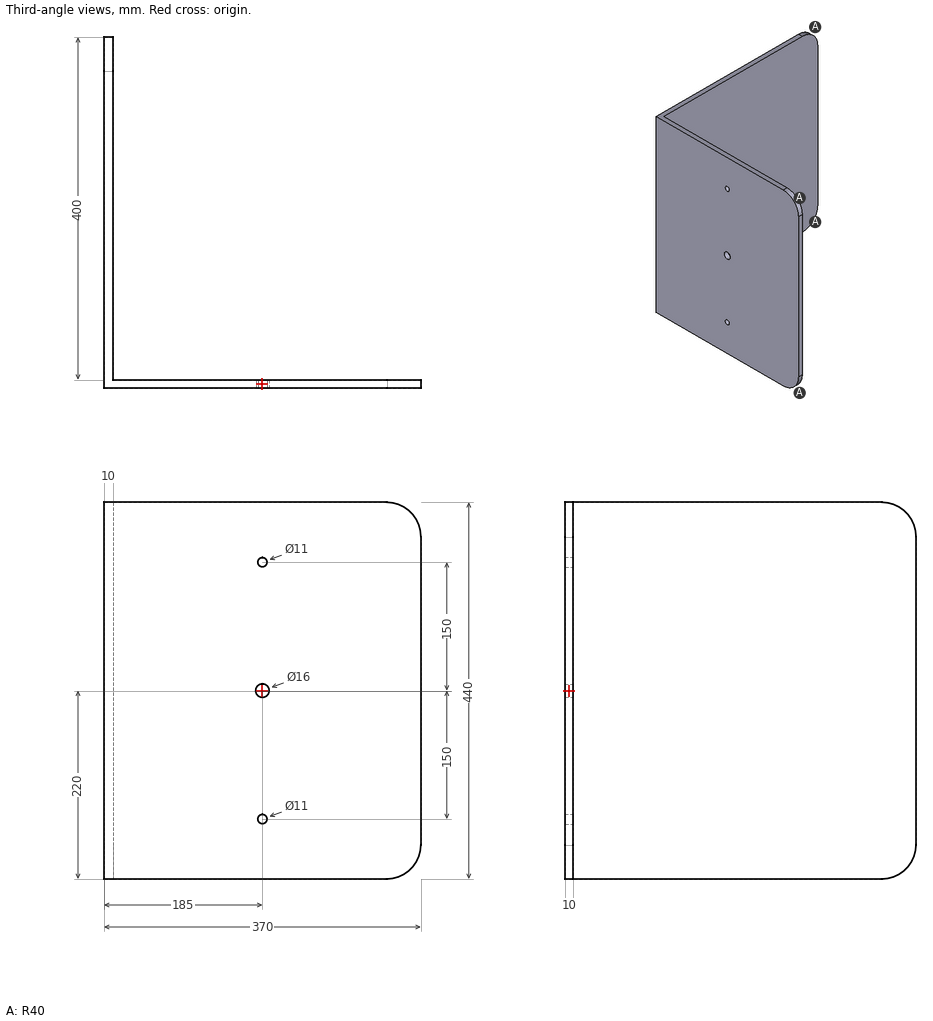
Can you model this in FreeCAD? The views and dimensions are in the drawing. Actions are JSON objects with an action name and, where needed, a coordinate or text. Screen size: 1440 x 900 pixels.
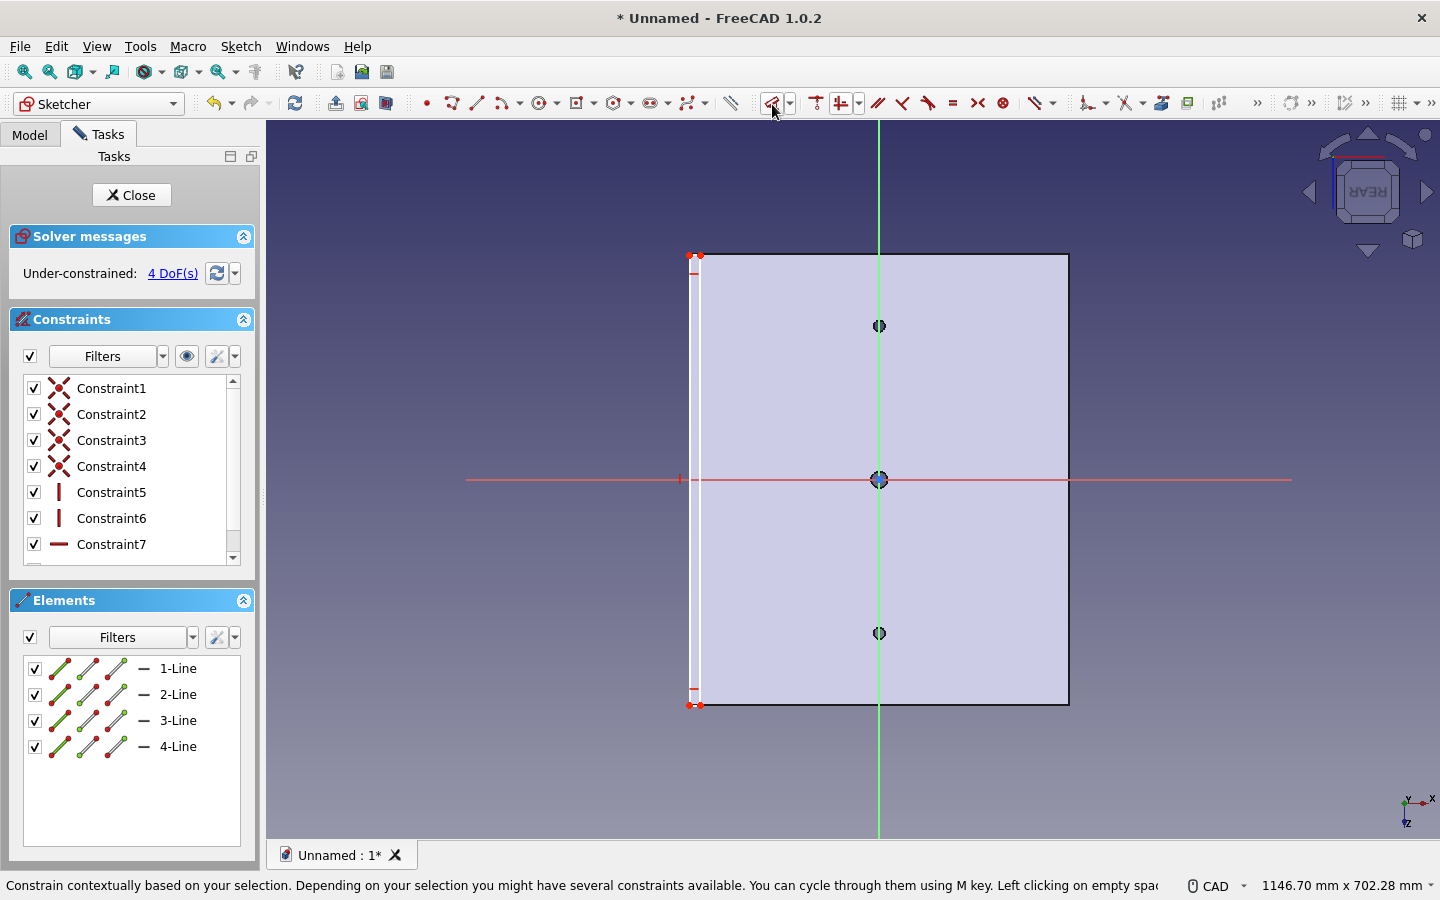
{"action": "scroll", "coordinate": [695, 706], "scroll_direction": "up", "scroll_amount": 7}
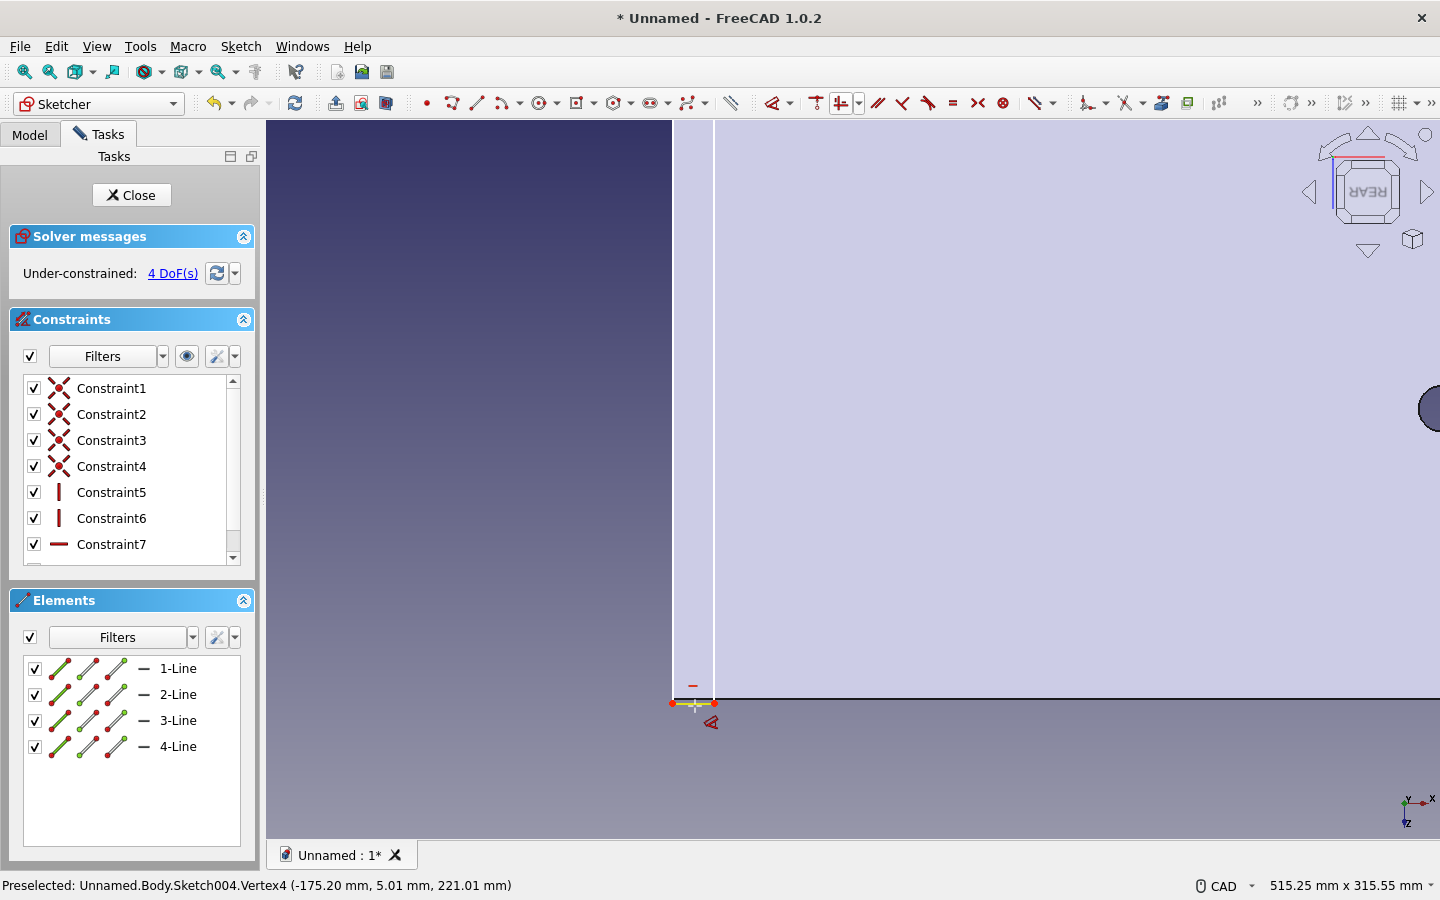
{"action": "left_click", "coordinate": [693, 704]}
{"action": "left_click", "coordinate": [693, 738]}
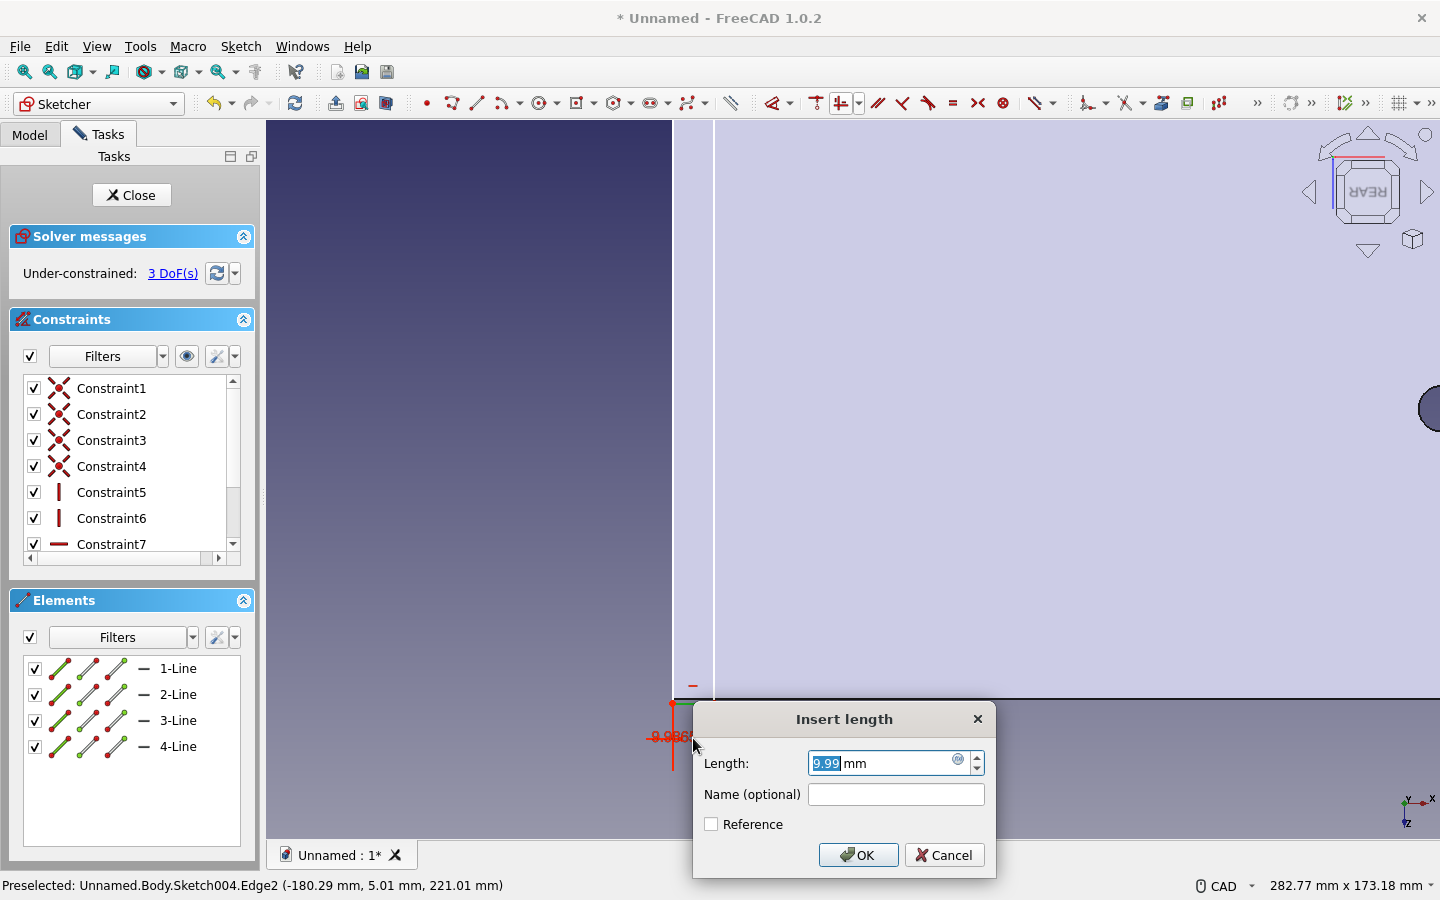
{"action": "type", "text": "10"}
{"action": "key", "text": "Return"}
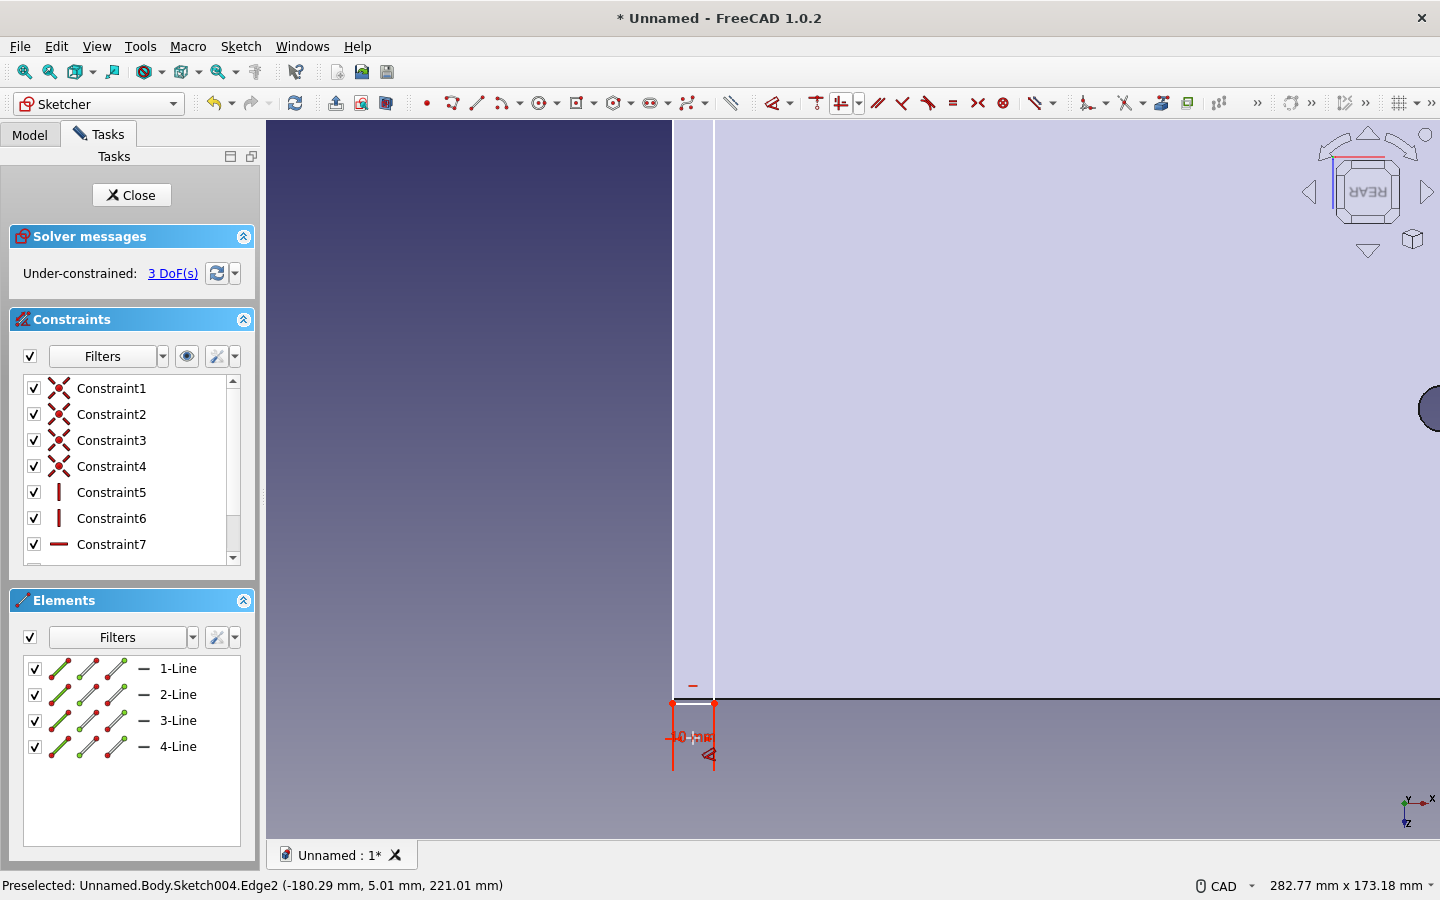
{"action": "left_click", "coordinate": [673, 155]}
{"action": "left_click", "coordinate": [639, 426]}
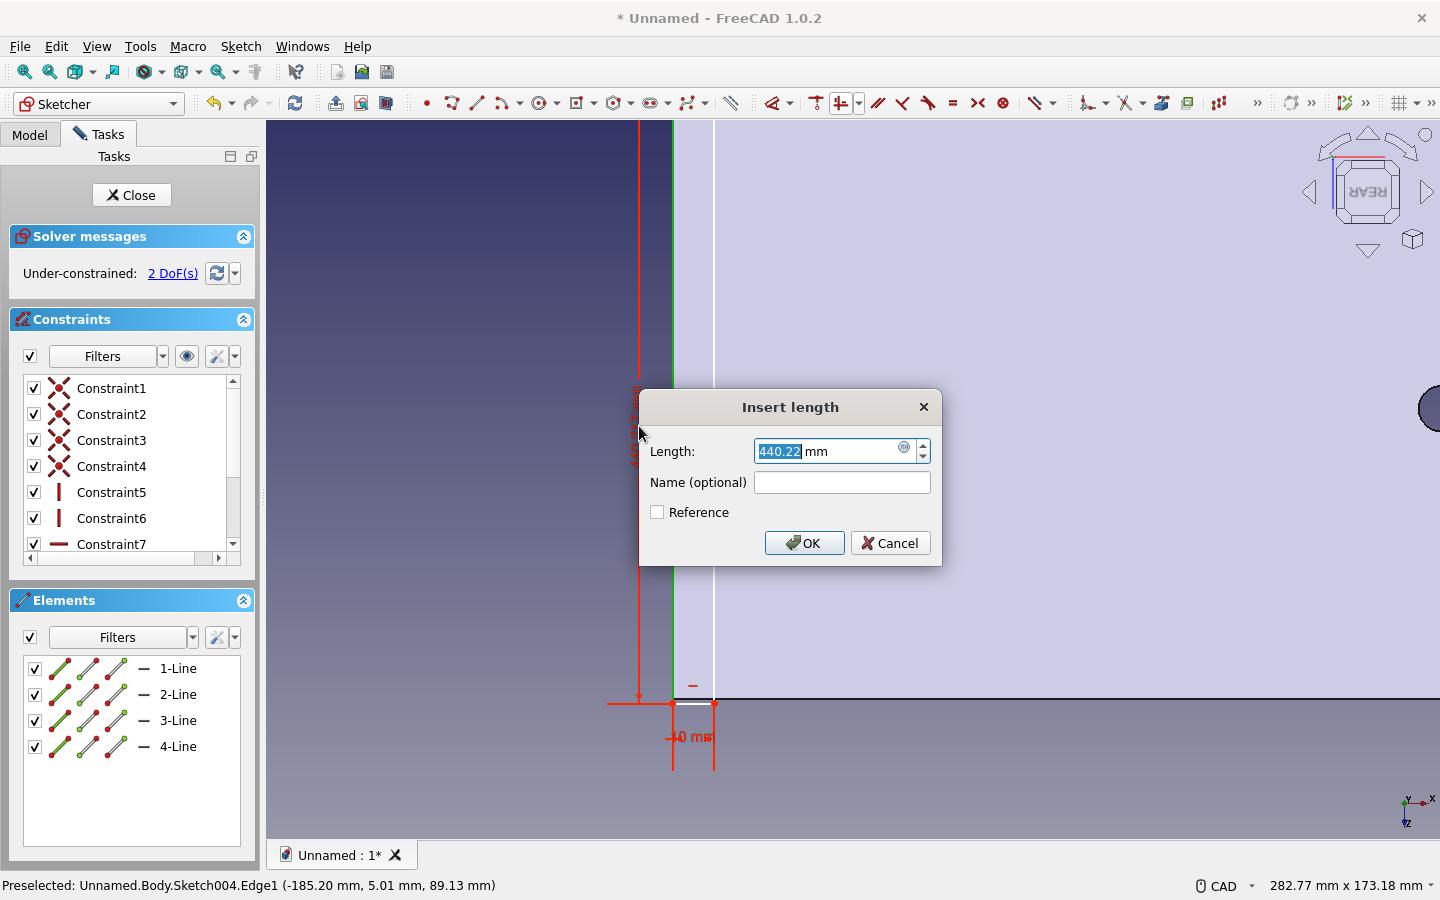
{"action": "type", "text": "440"}
{"action": "key", "text": "Return"}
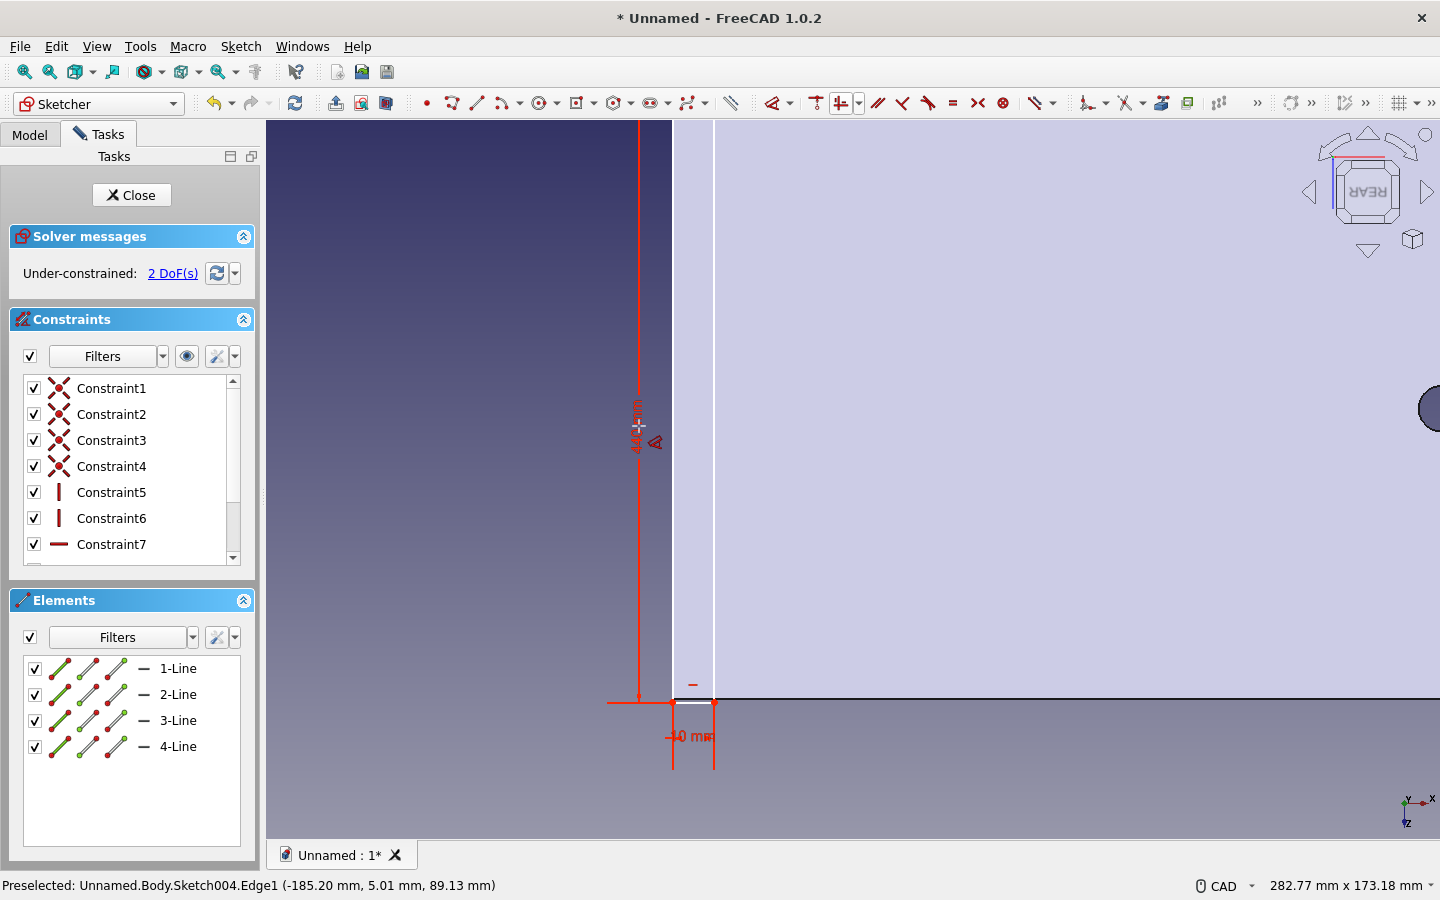
{"action": "scroll", "coordinate": [695, 707], "scroll_direction": "down", "scroll_amount": 7}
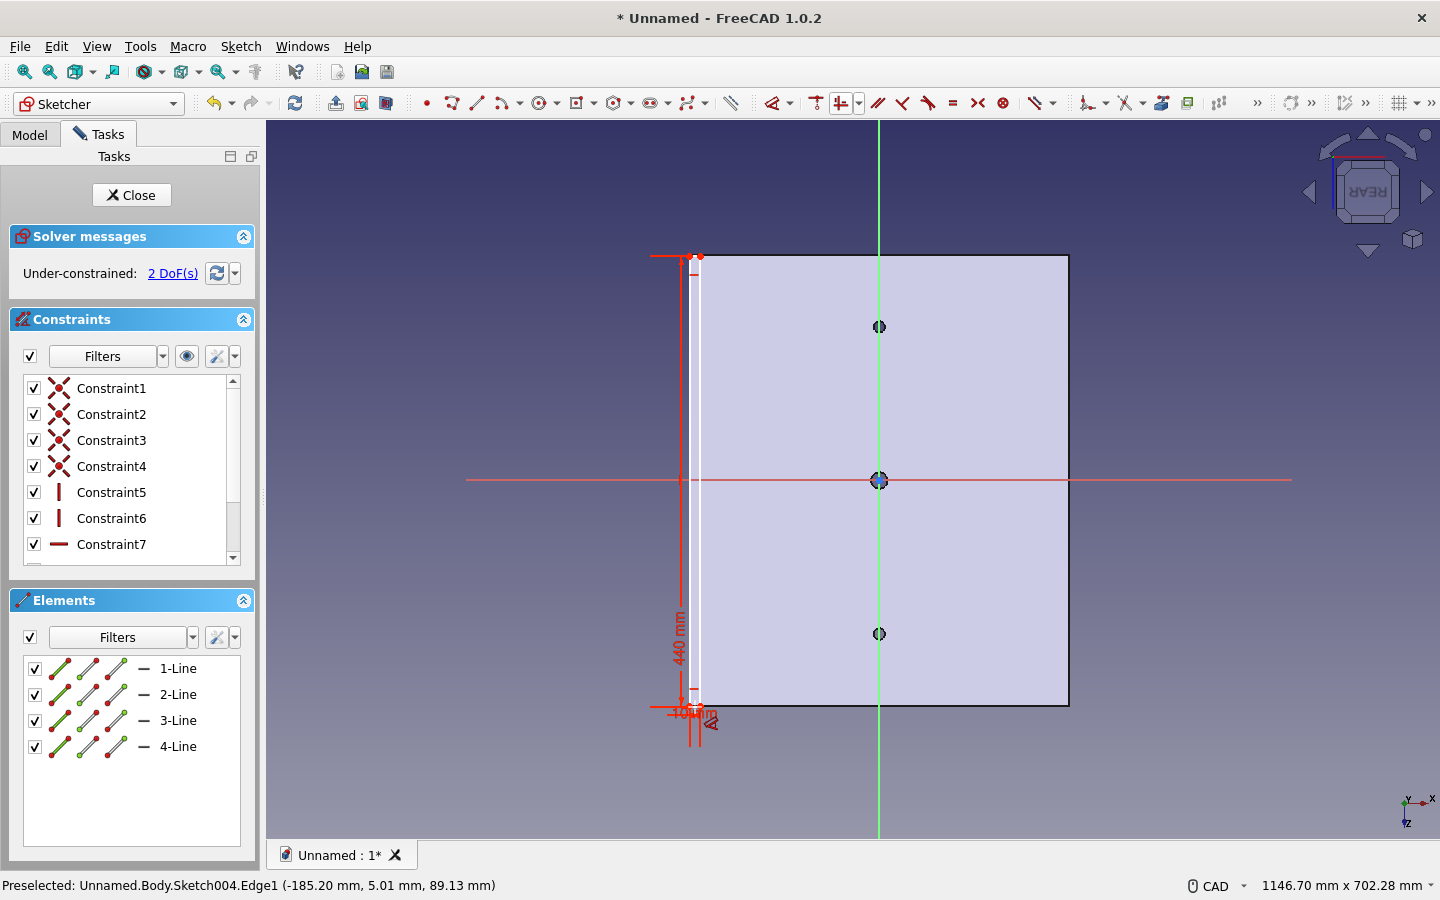
{"action": "left_click", "coordinate": [690, 256]}
{"action": "left_click", "coordinate": [785, 222]}